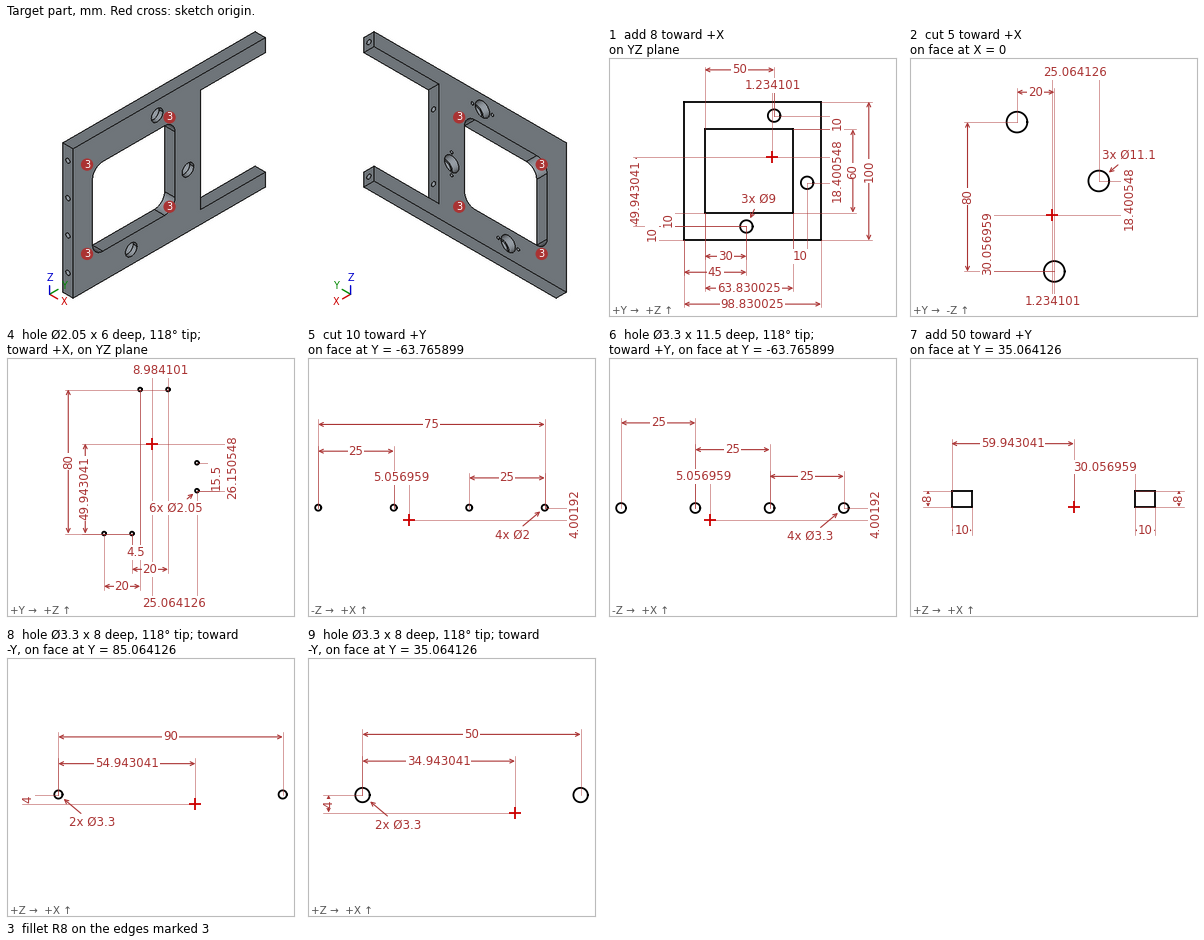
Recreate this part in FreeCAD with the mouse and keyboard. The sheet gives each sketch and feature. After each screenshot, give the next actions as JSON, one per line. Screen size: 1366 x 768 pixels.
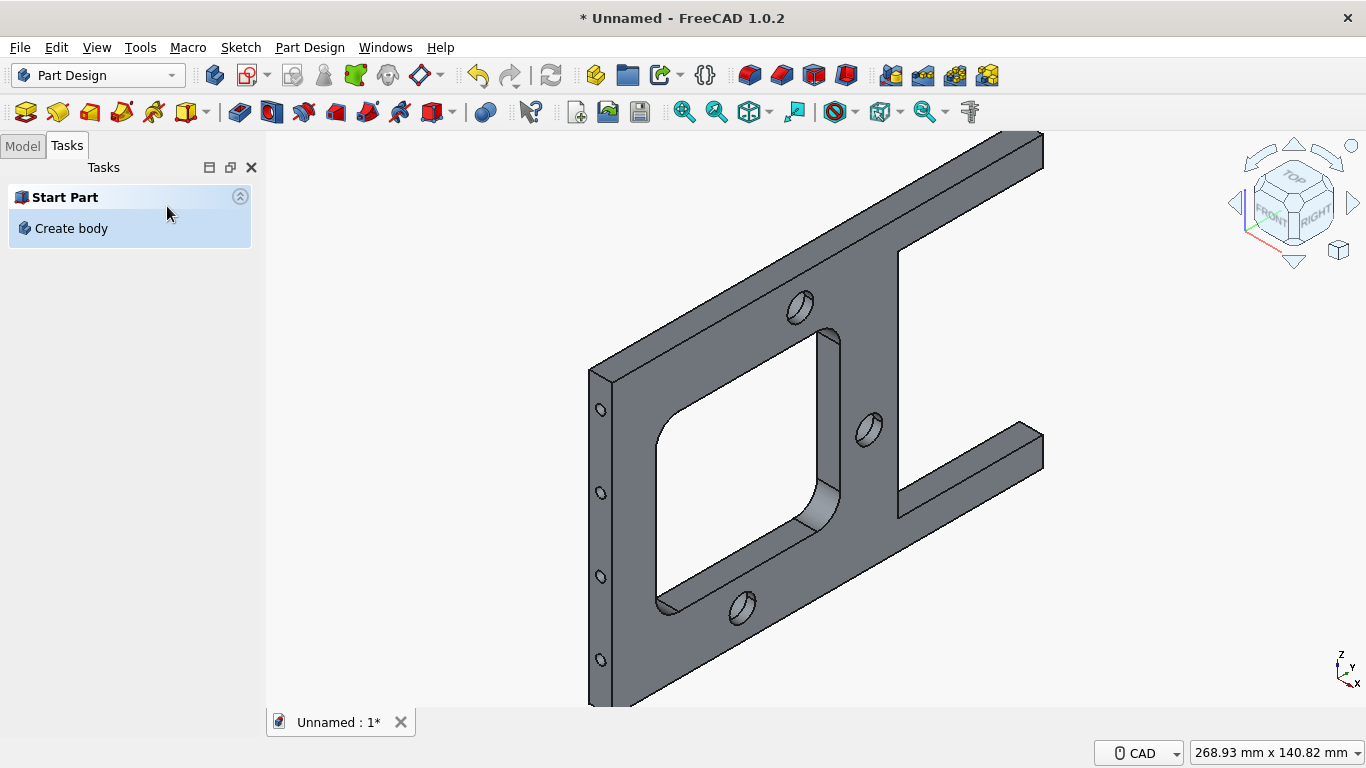
{"action": "key", "text": "v f"}